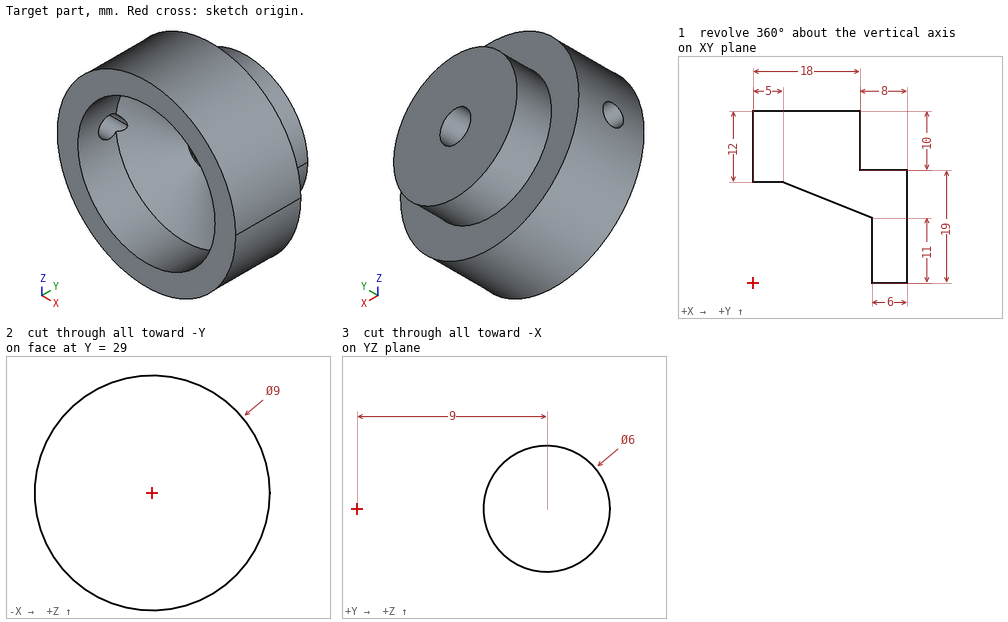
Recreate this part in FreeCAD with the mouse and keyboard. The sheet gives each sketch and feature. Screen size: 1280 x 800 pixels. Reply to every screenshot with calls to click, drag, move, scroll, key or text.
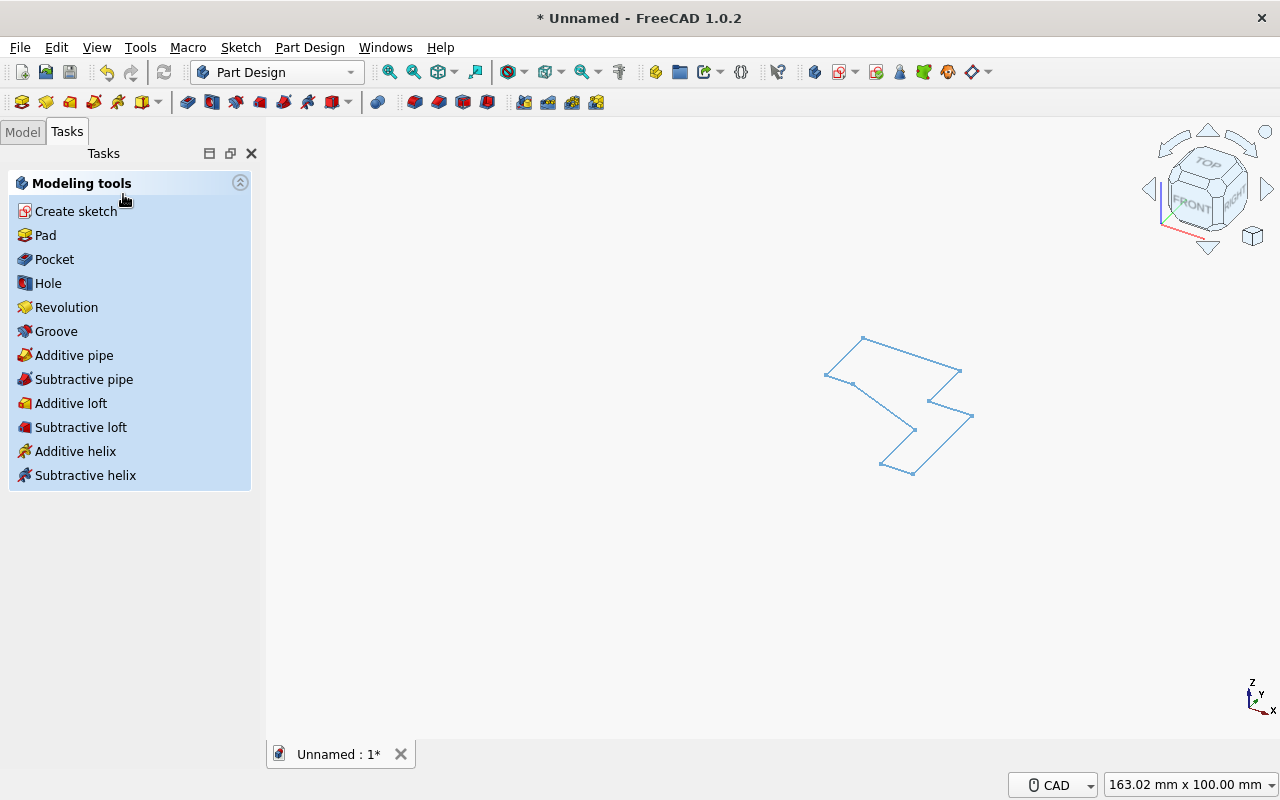
click(46, 102)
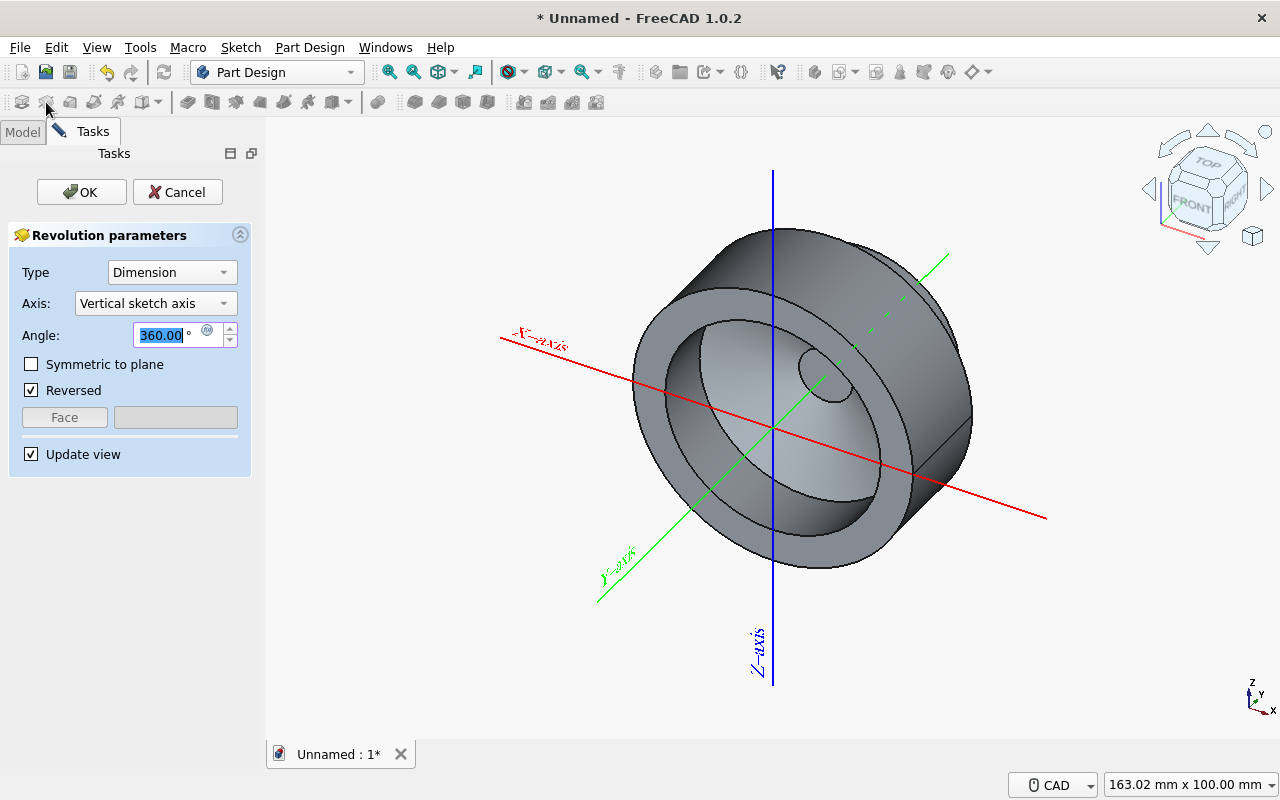
click(82, 192)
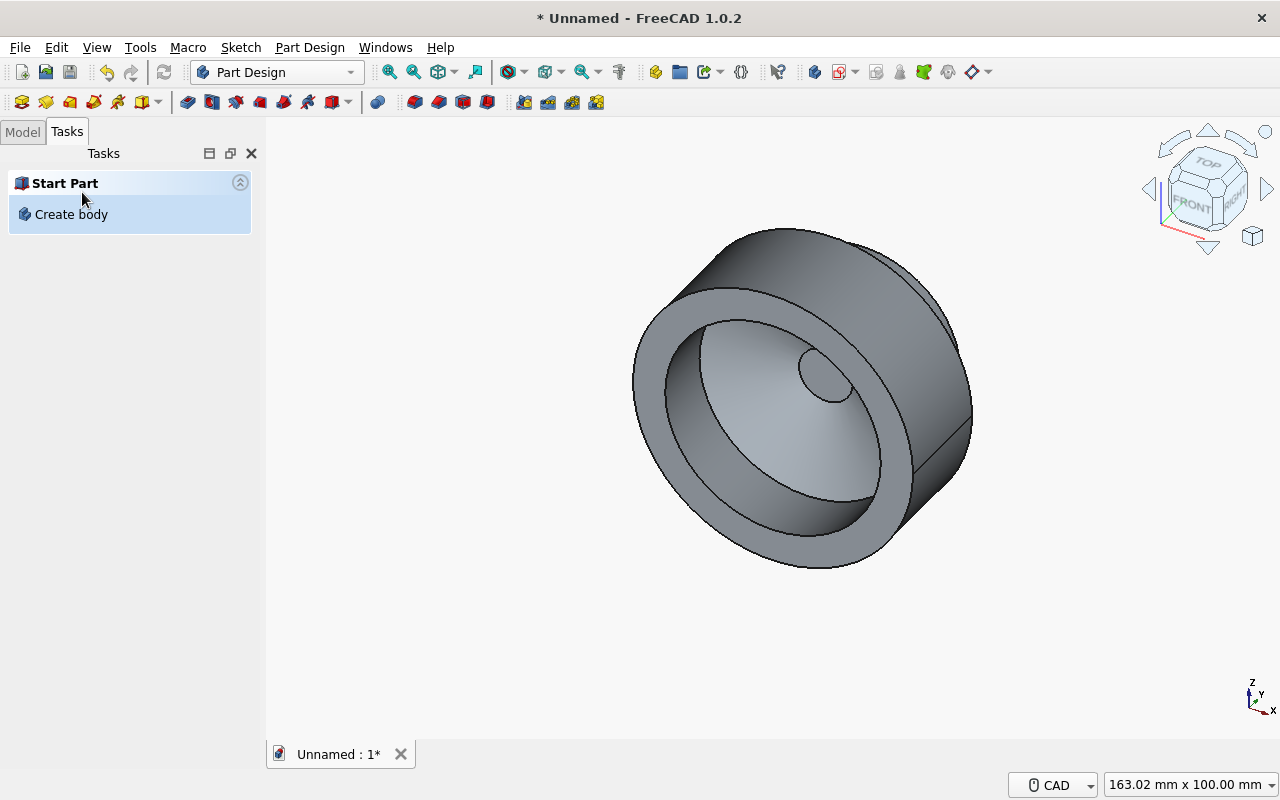
key(4)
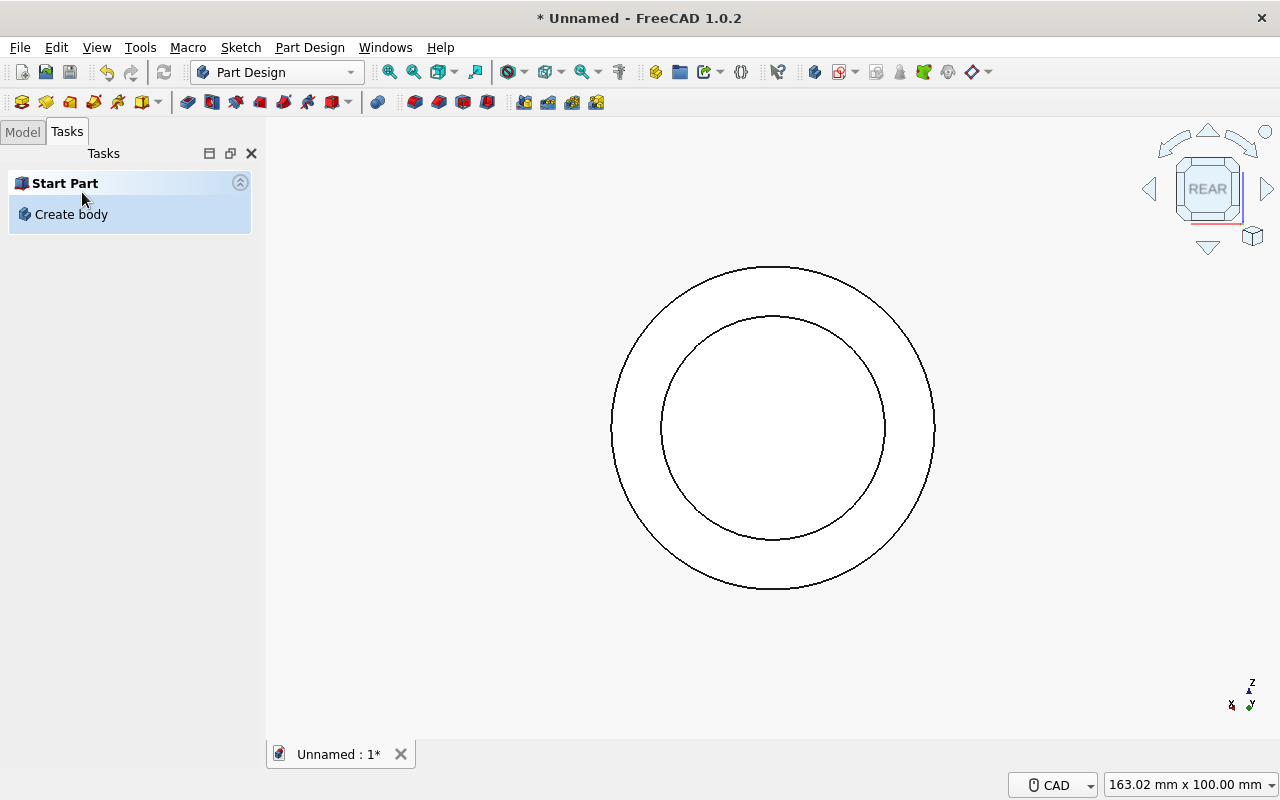
click(773, 427)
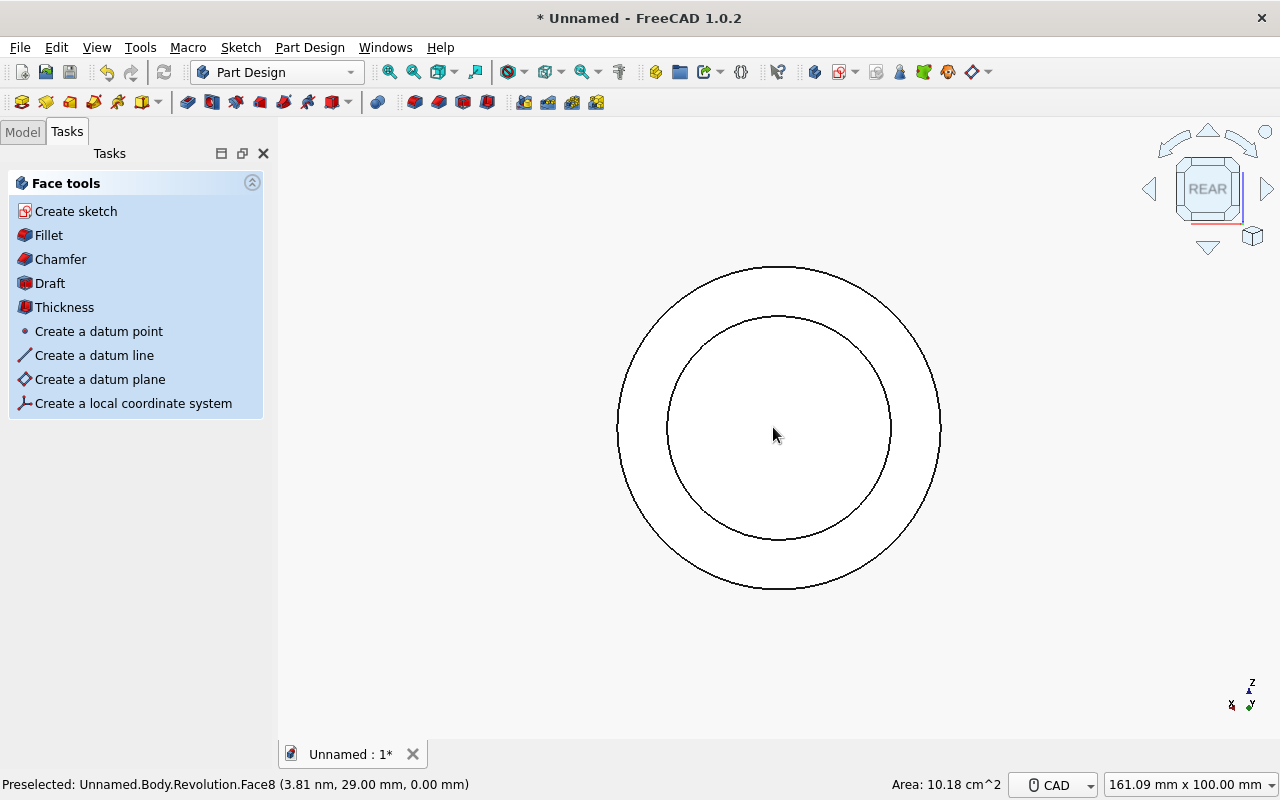
click(840, 72)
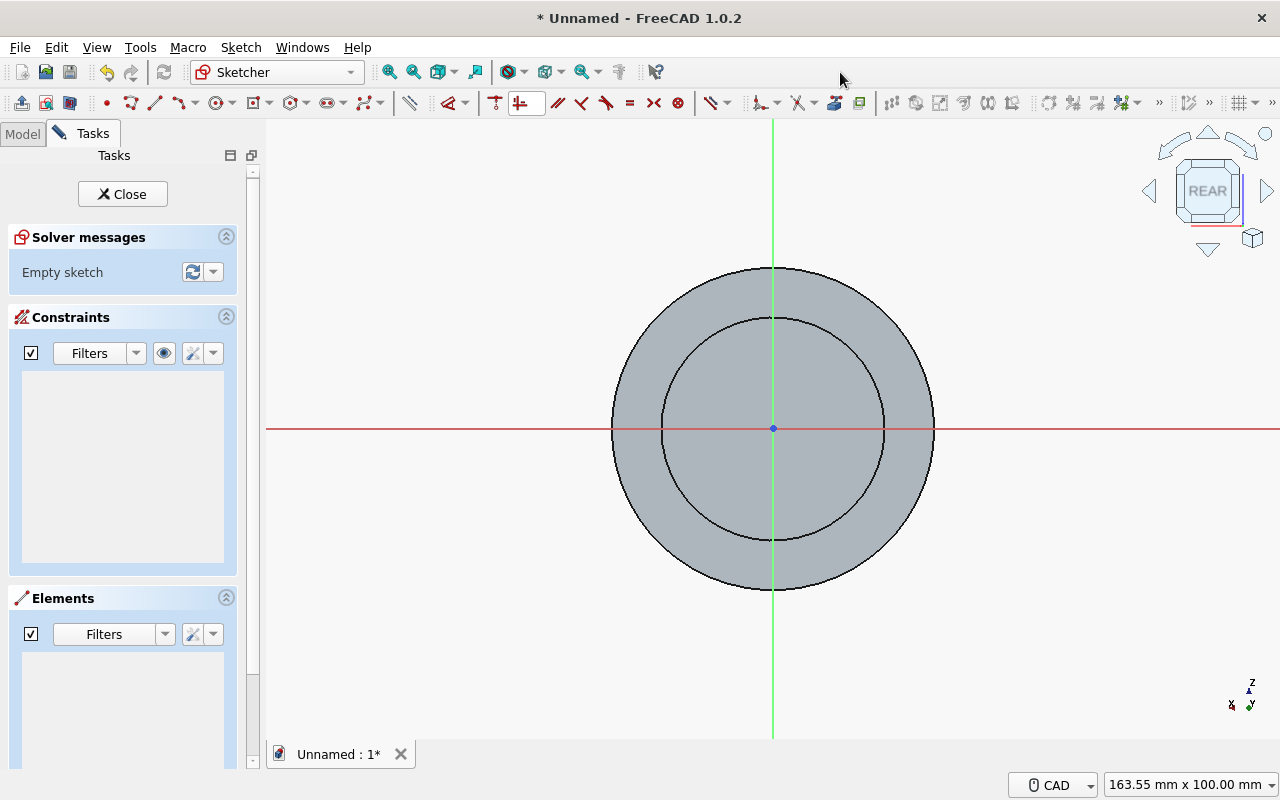
scroll(784, 429, up, 10)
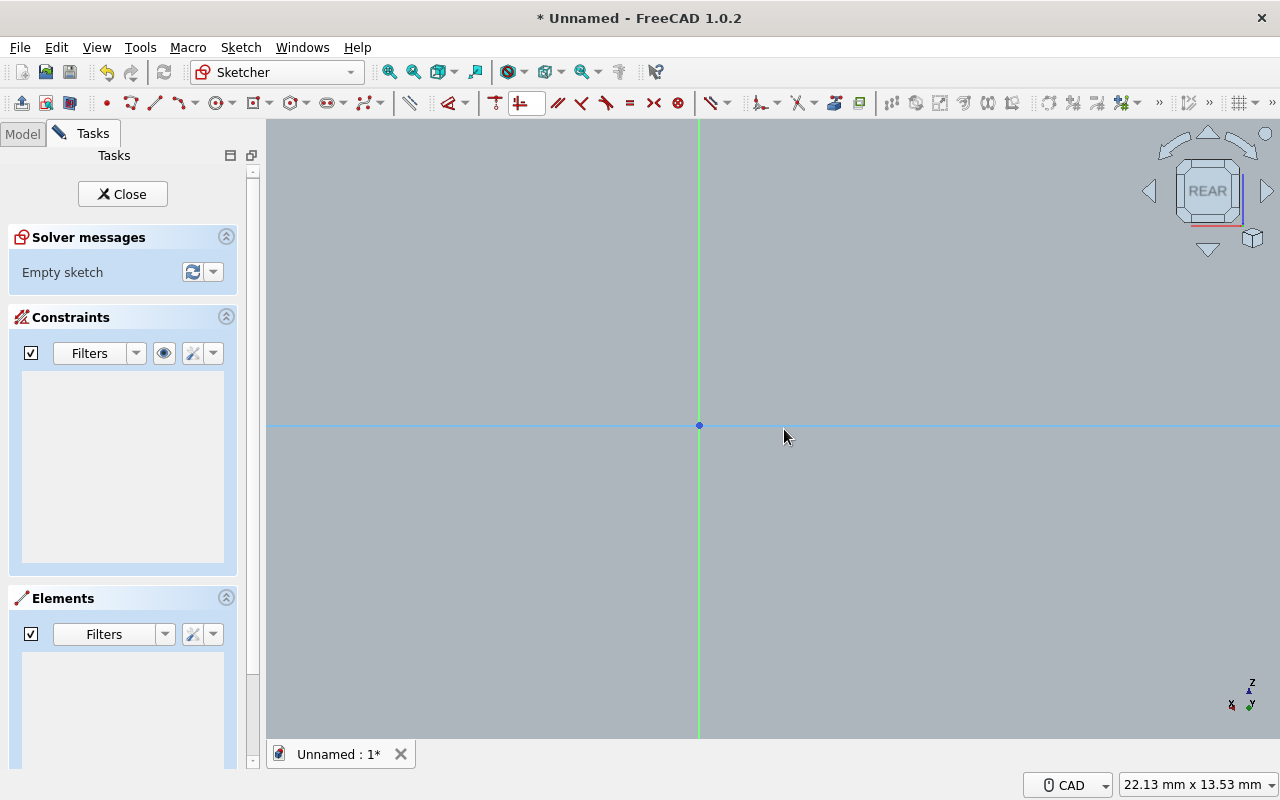
click(216, 104)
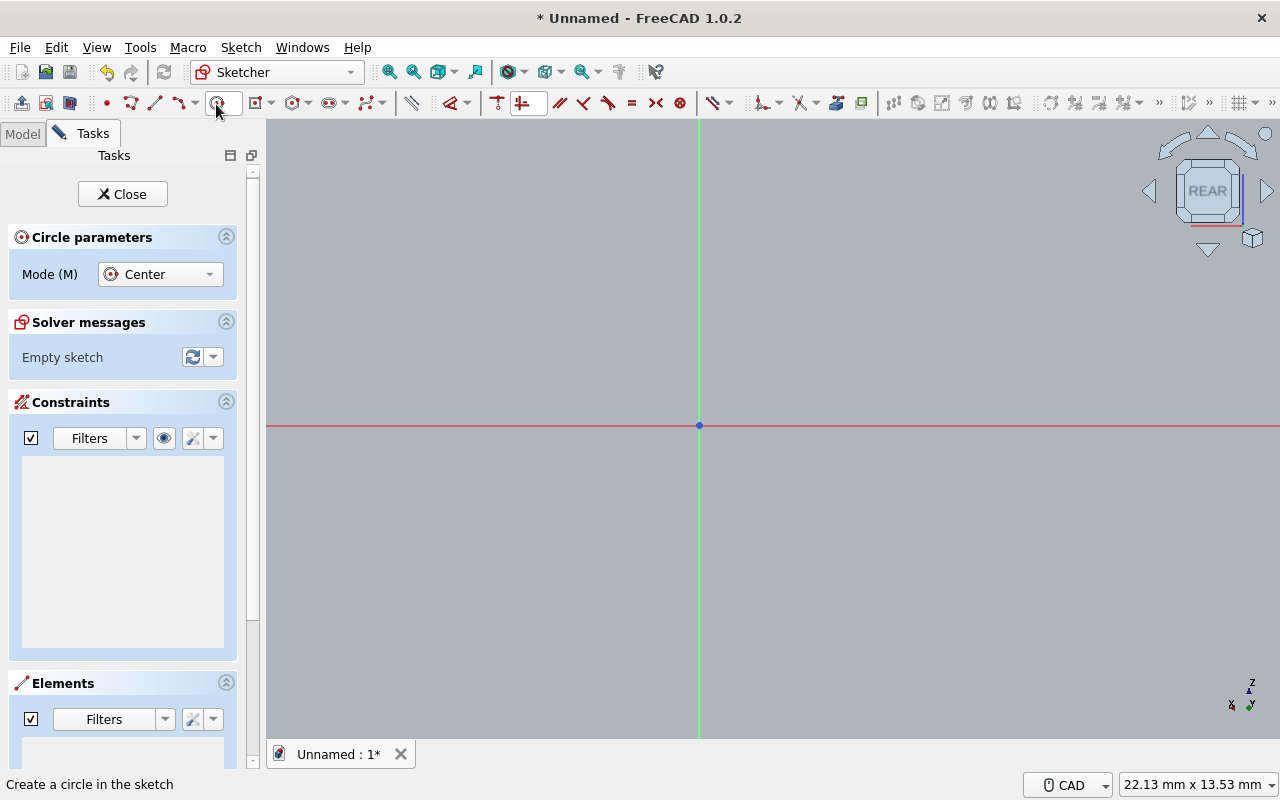
click(699, 426)
click(845, 280)
key(Escape)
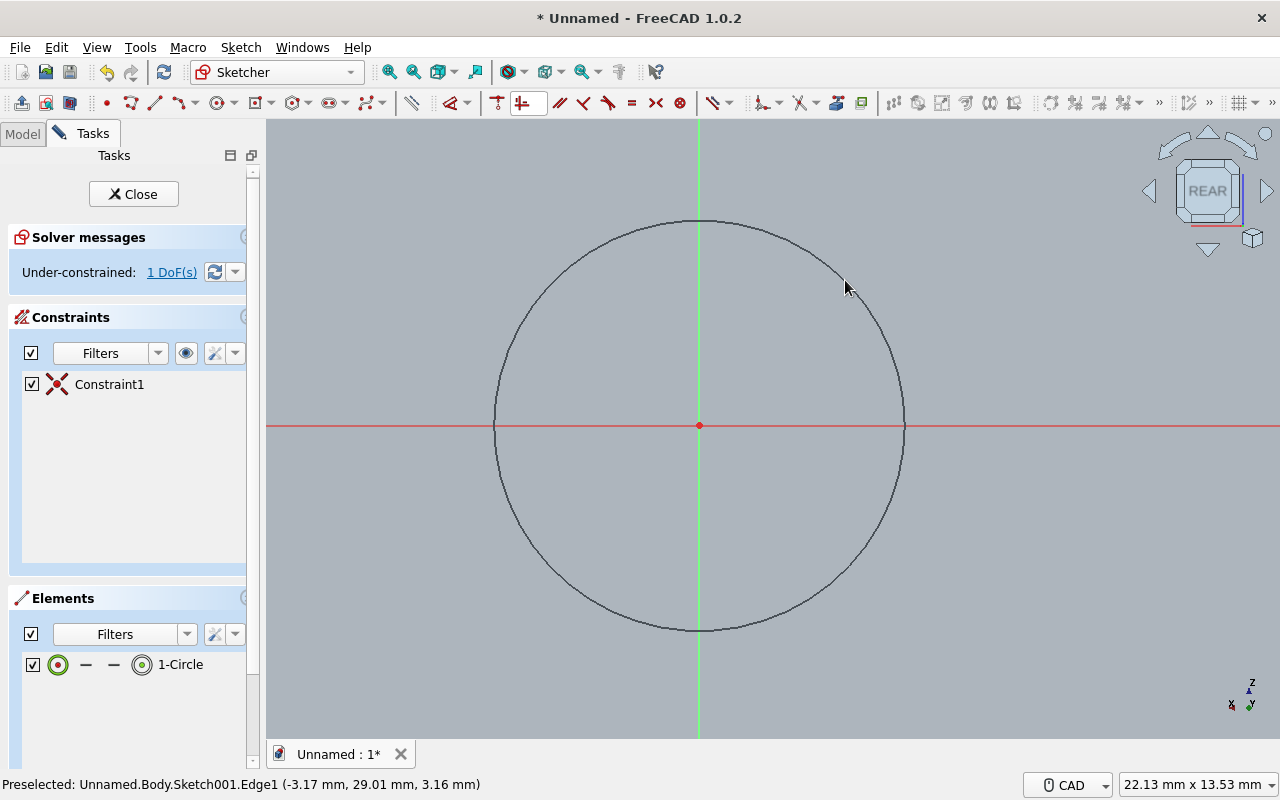
click(450, 104)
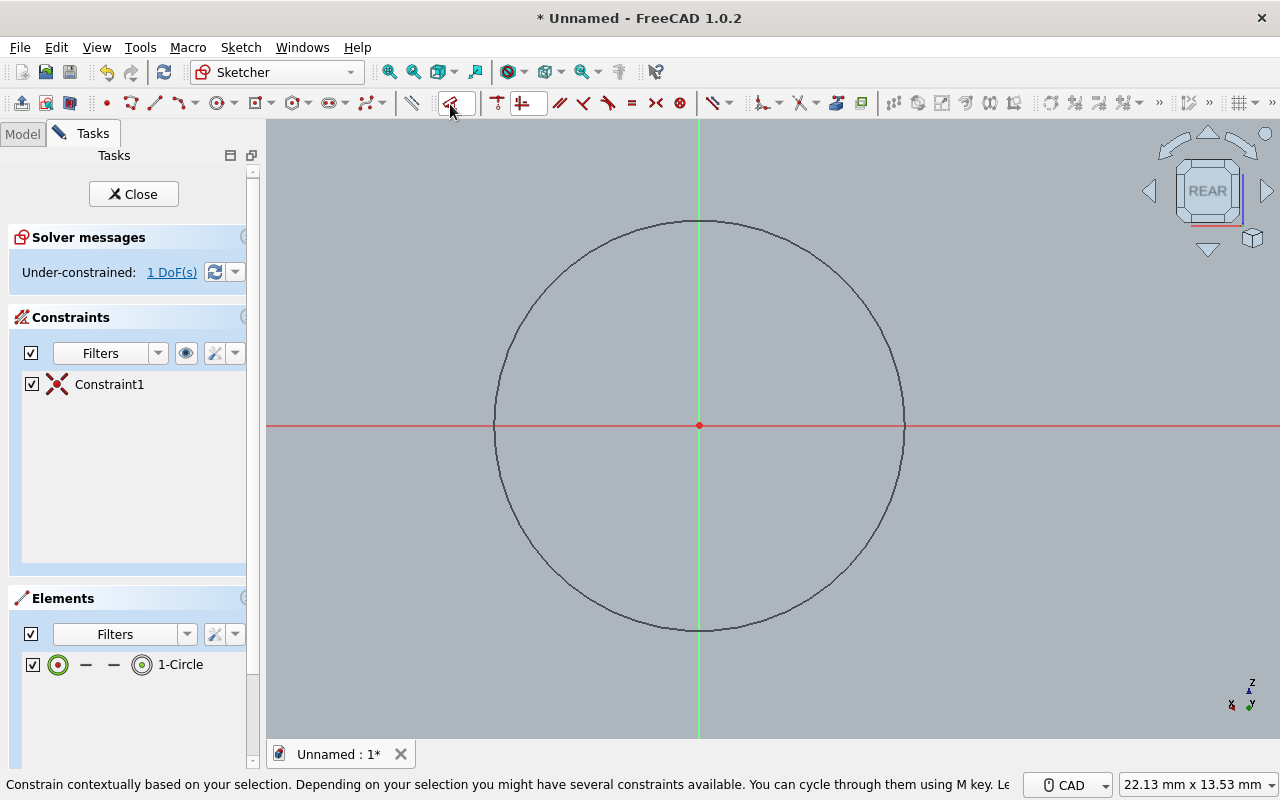
click(844, 280)
click(867, 257)